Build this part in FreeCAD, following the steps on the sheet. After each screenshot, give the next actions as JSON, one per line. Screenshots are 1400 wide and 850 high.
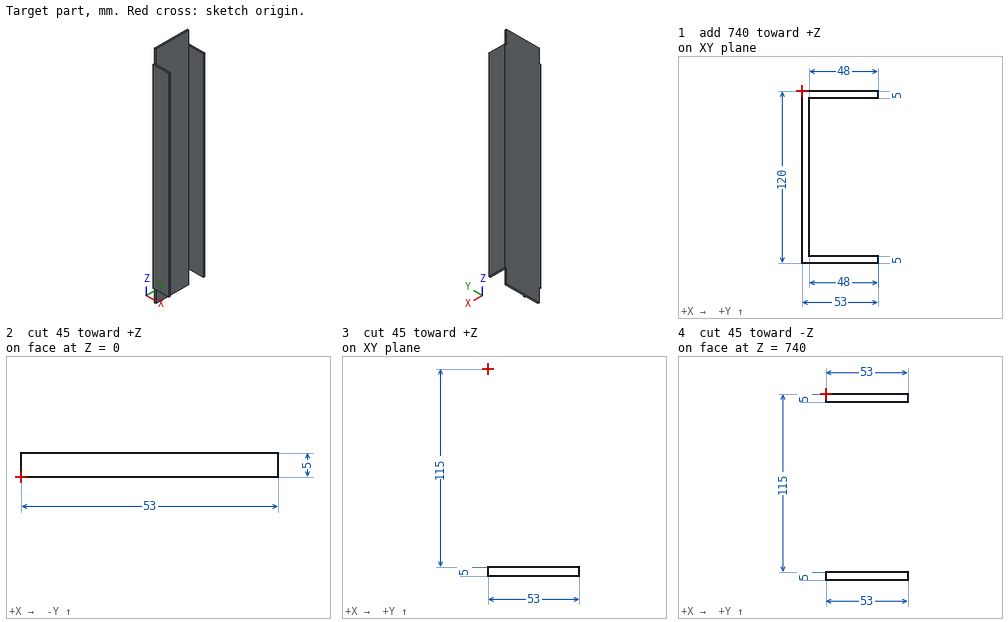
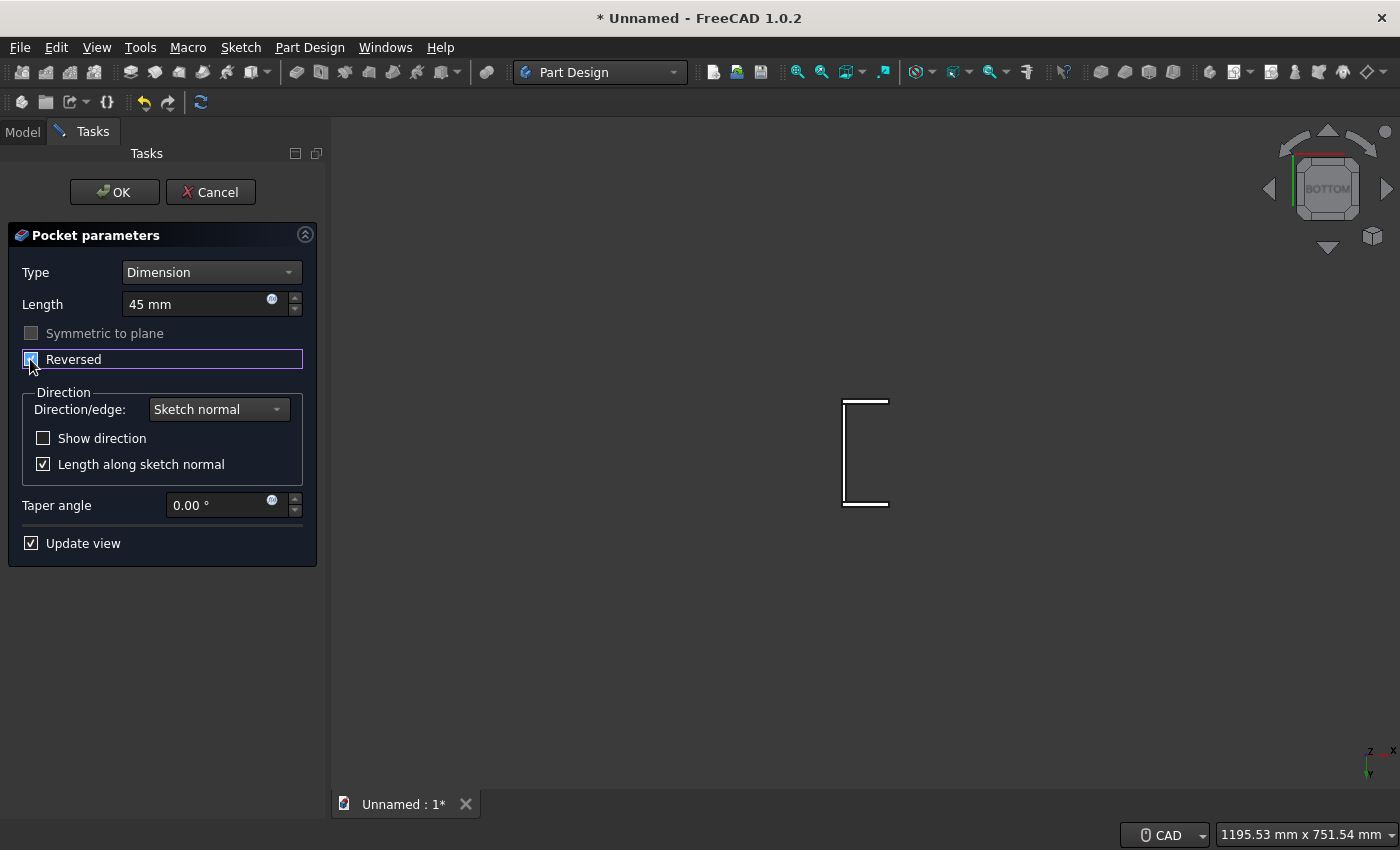
{"action": "left_click", "coordinate": [115, 192]}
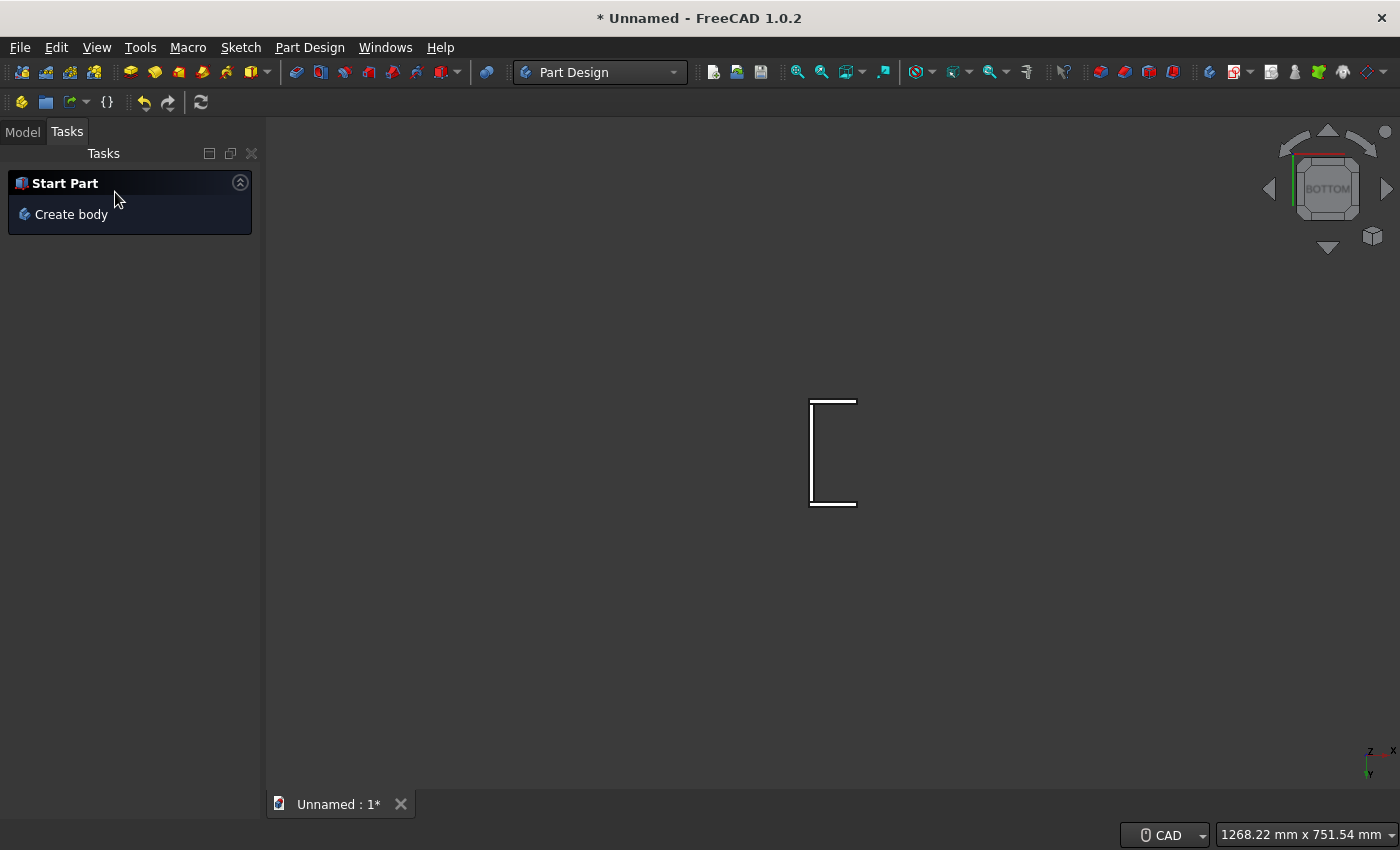
{"action": "left_click", "coordinate": [798, 72]}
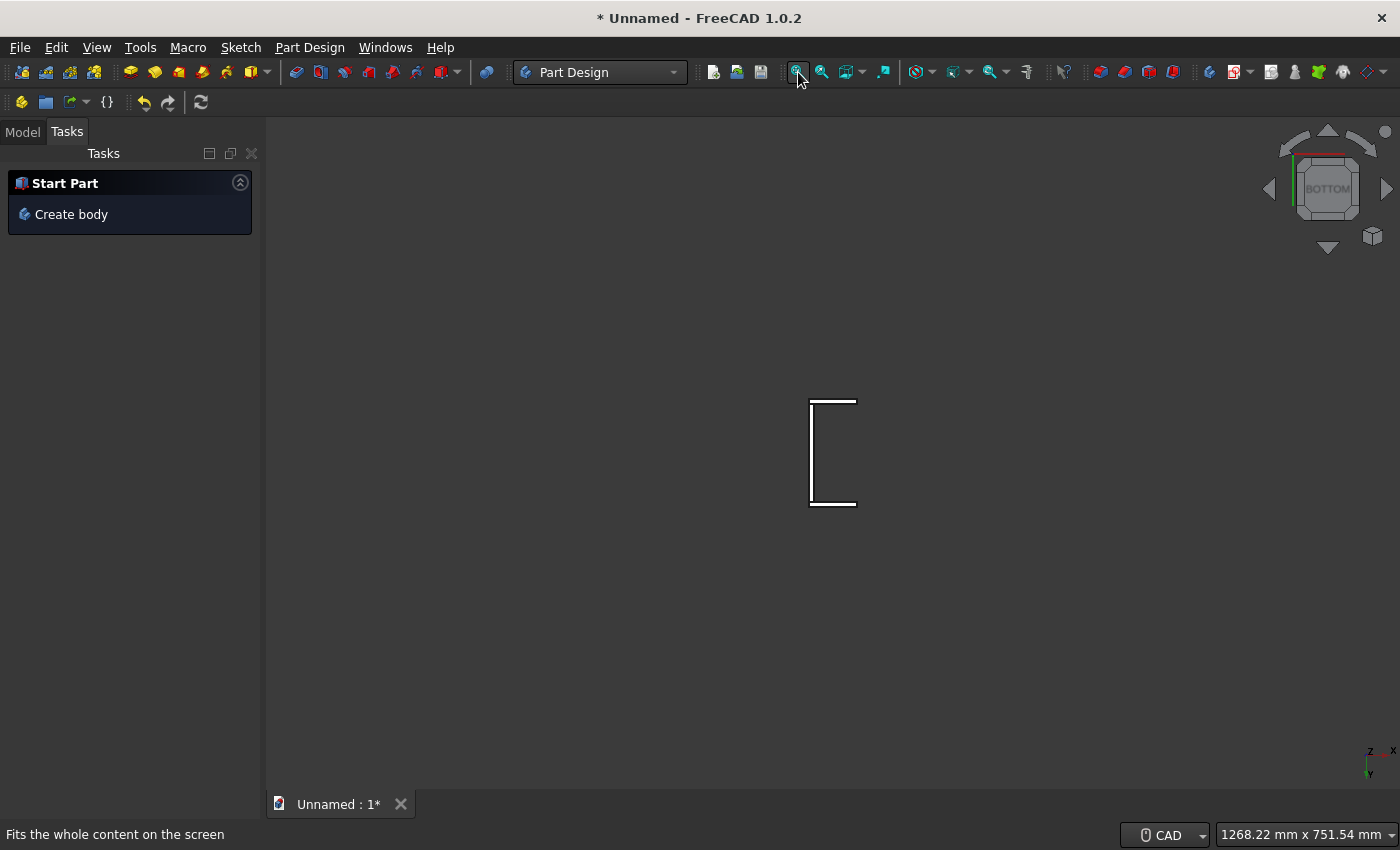
{"action": "key", "text": "0"}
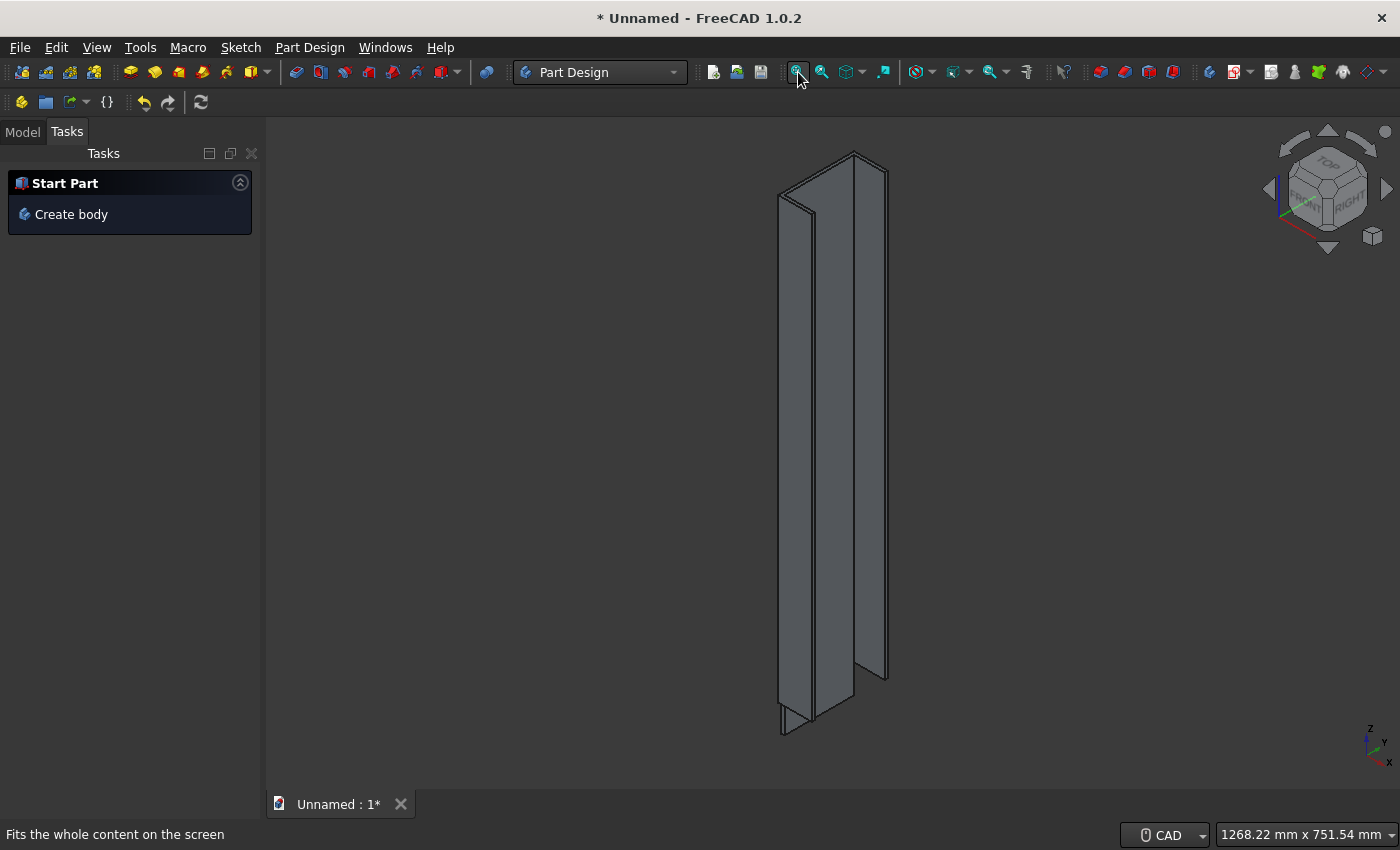
{"action": "scroll", "coordinate": [851, 155], "scroll_direction": "up", "scroll_amount": 13}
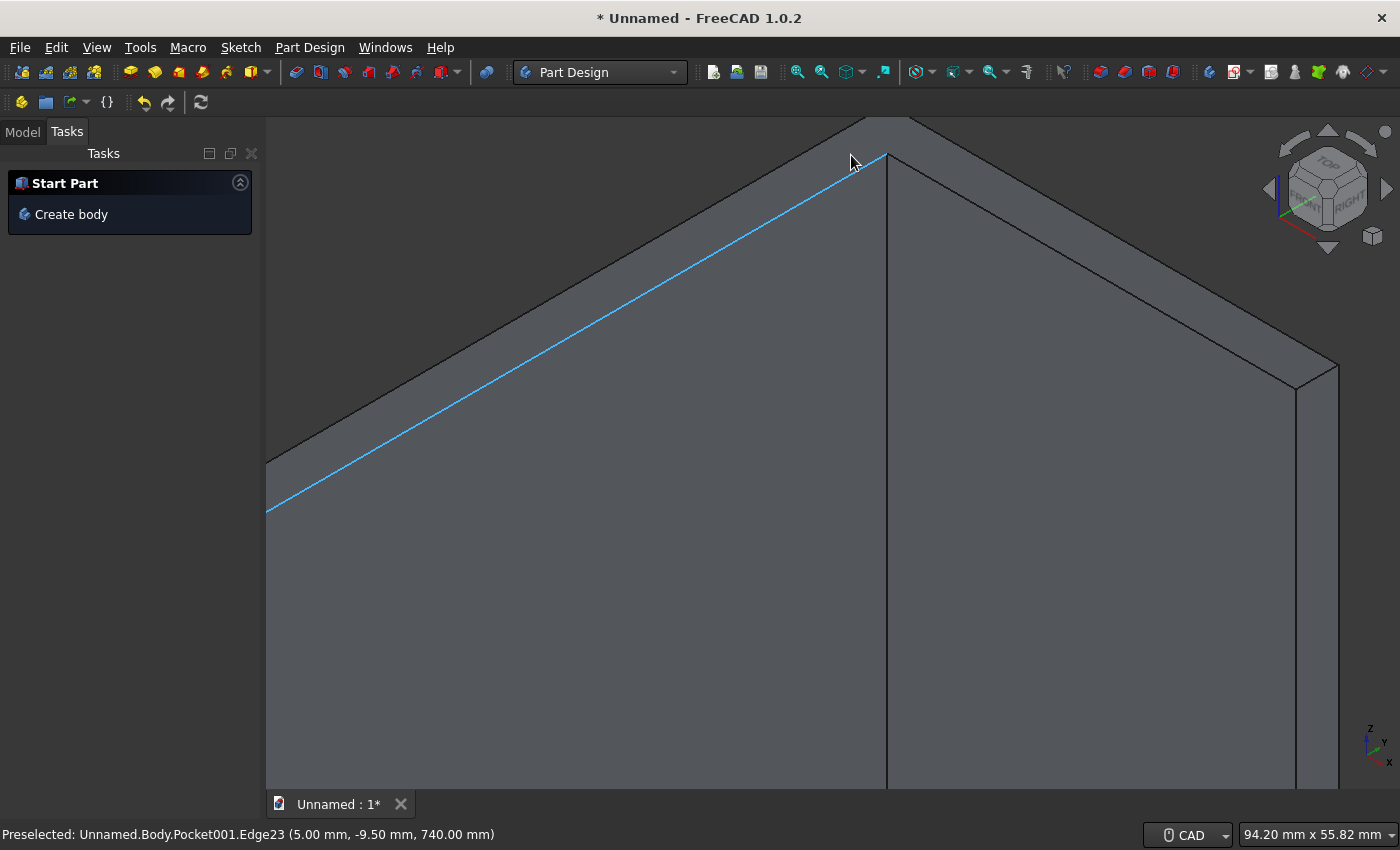
{"action": "left_click", "coordinate": [847, 164]}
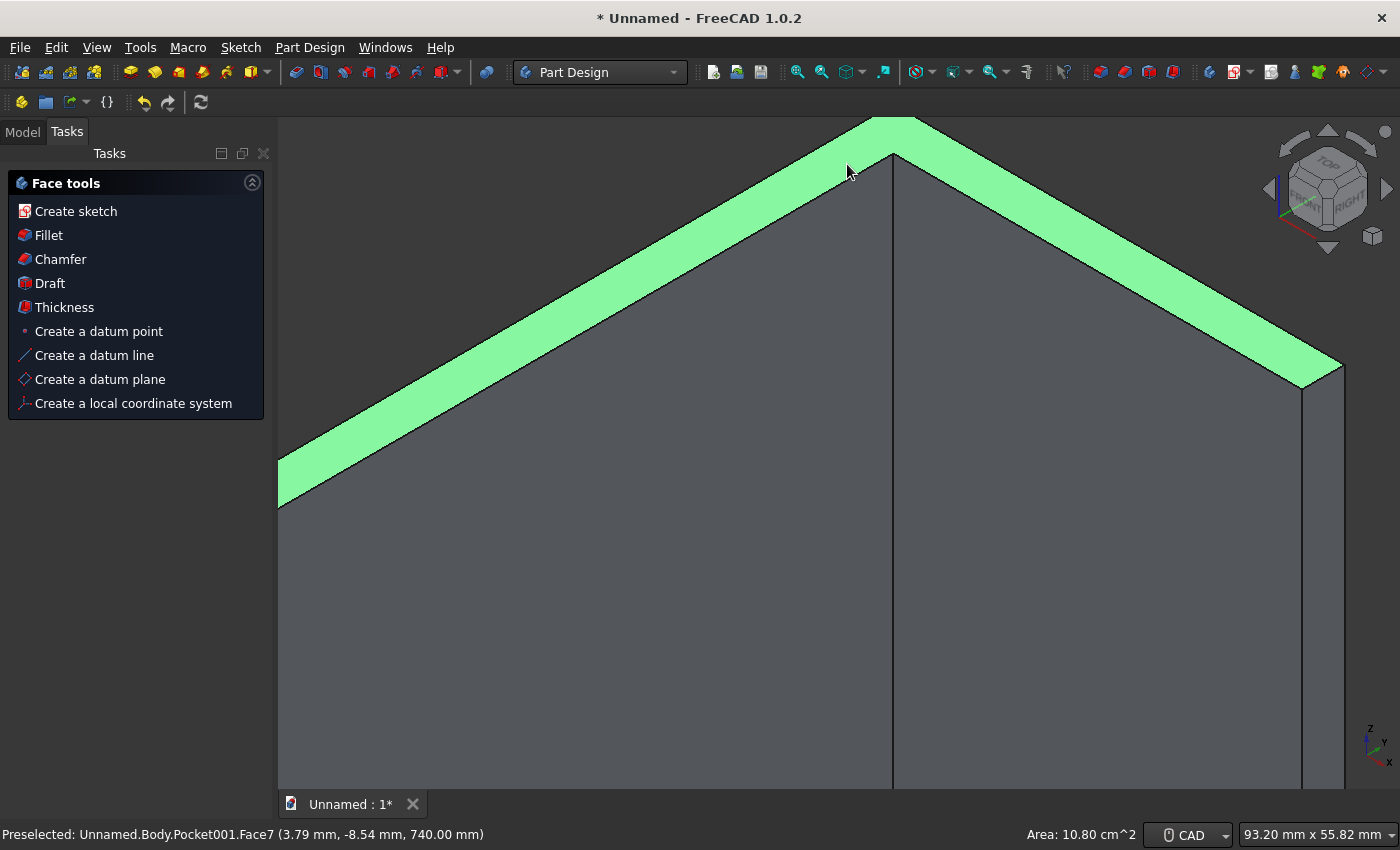
{"action": "left_click", "coordinate": [1234, 72]}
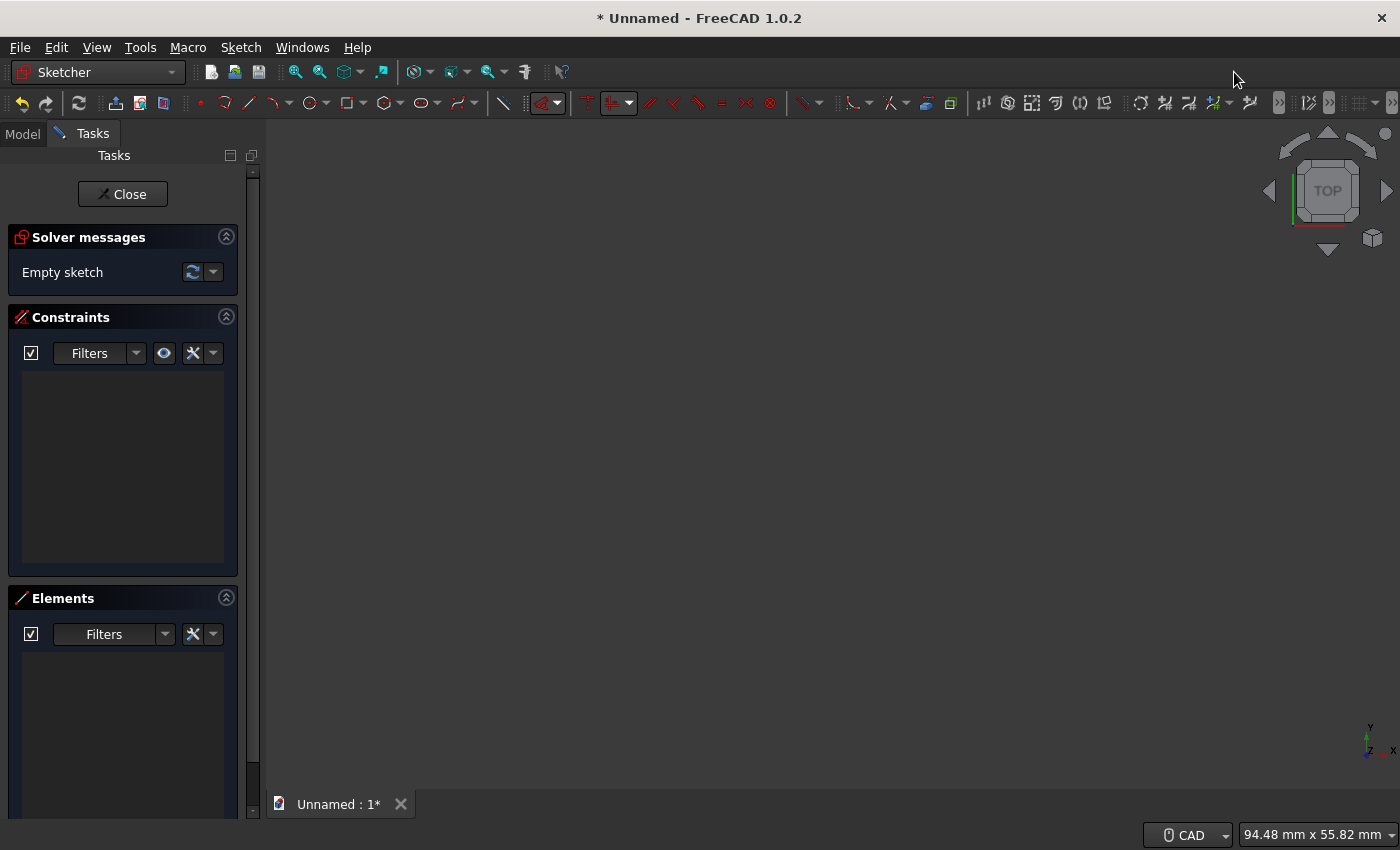
{"action": "scroll", "coordinate": [406, 147], "scroll_direction": "down", "scroll_amount": 8}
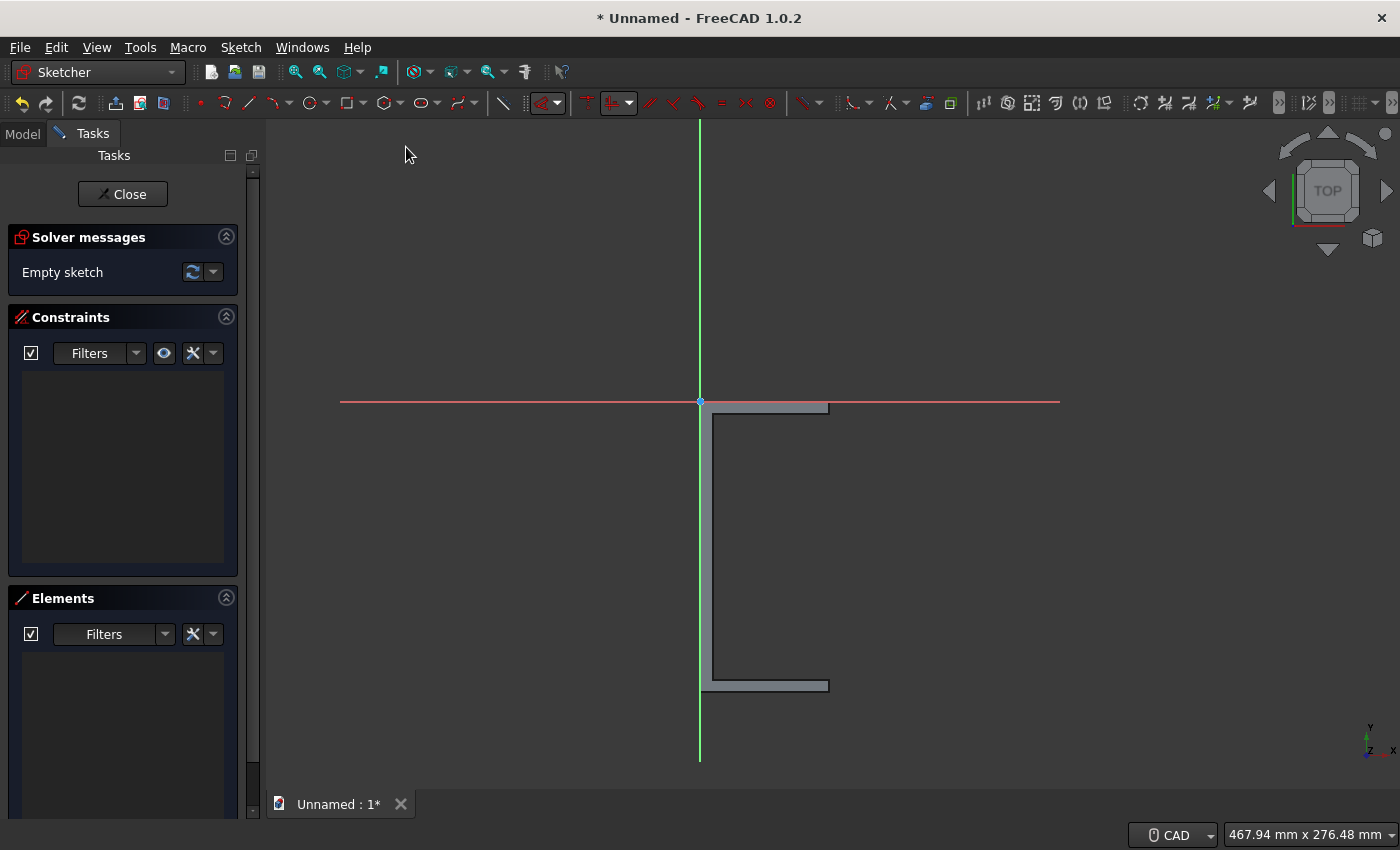
{"action": "scroll", "coordinate": [765, 736], "scroll_direction": "up", "scroll_amount": 2}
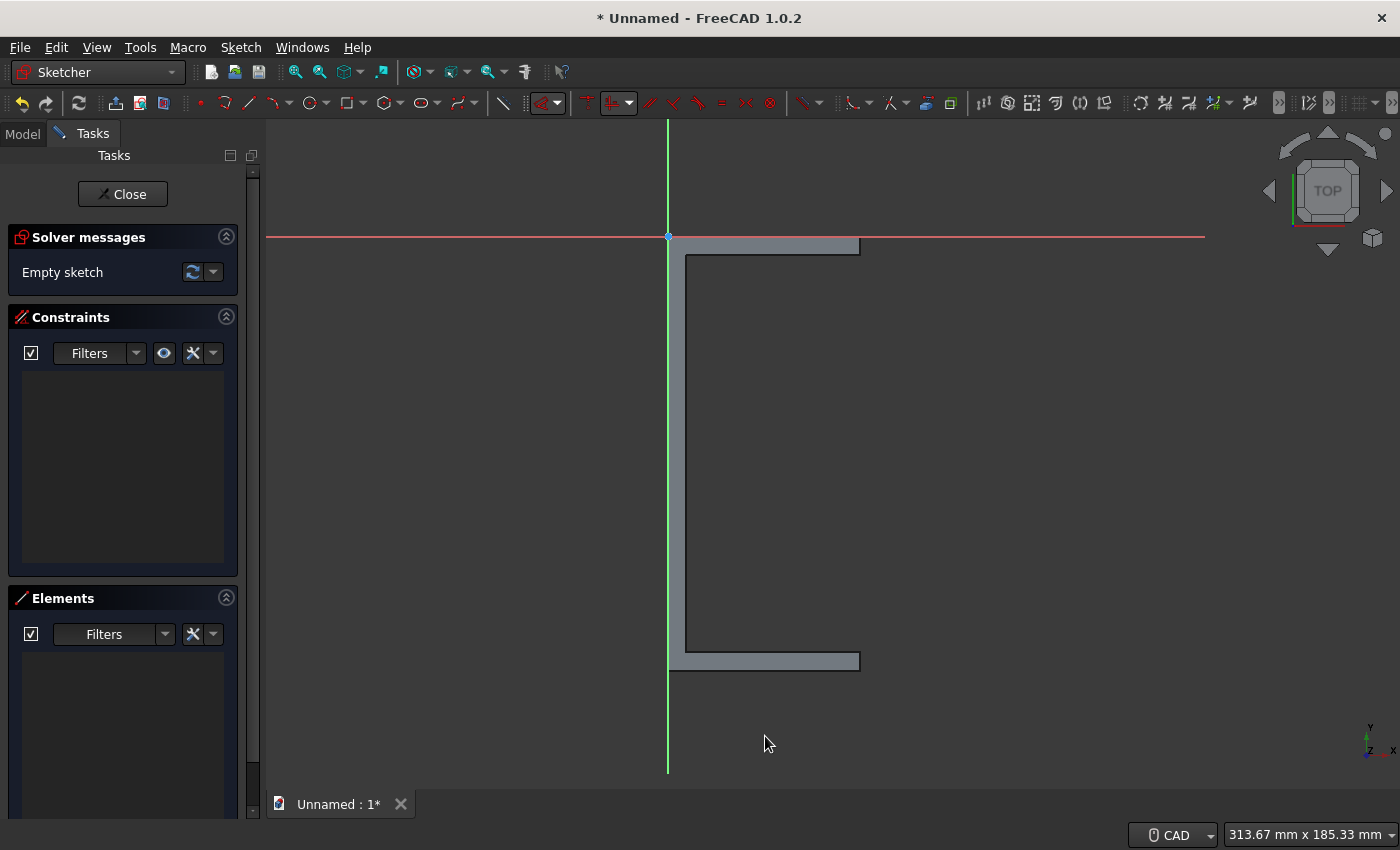
{"action": "left_click", "coordinate": [348, 104]}